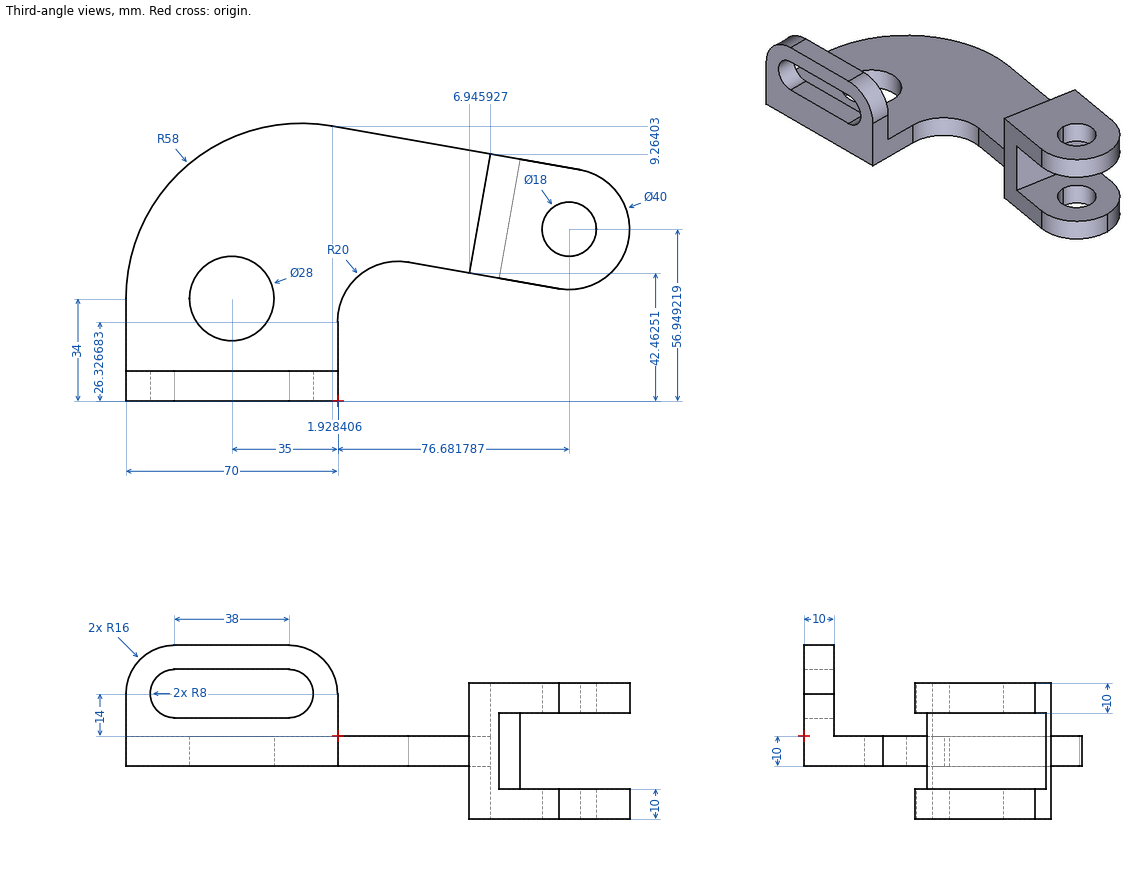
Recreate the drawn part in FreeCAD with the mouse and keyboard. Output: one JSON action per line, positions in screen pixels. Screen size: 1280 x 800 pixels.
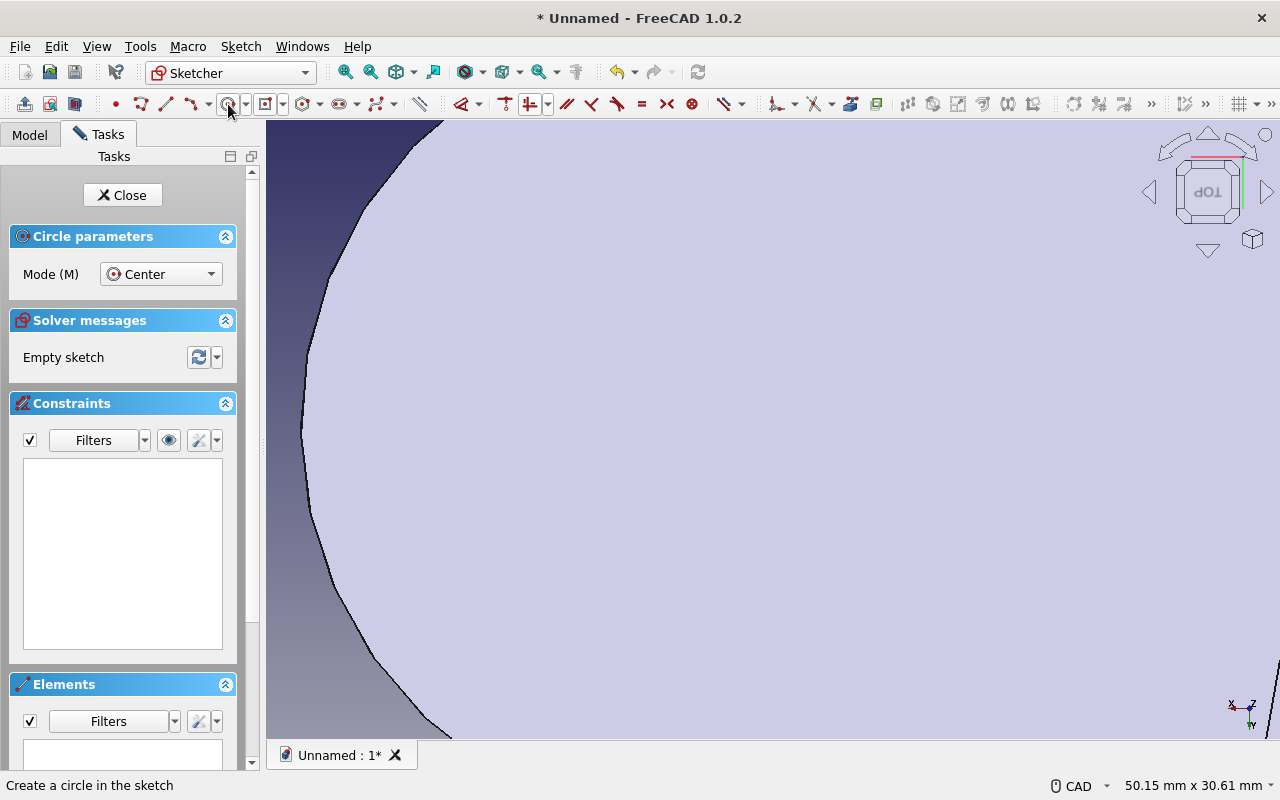
{"action": "left_click", "coordinate": [705, 426]}
{"action": "left_click", "coordinate": [834, 297]}
{"action": "key", "text": "Escape"}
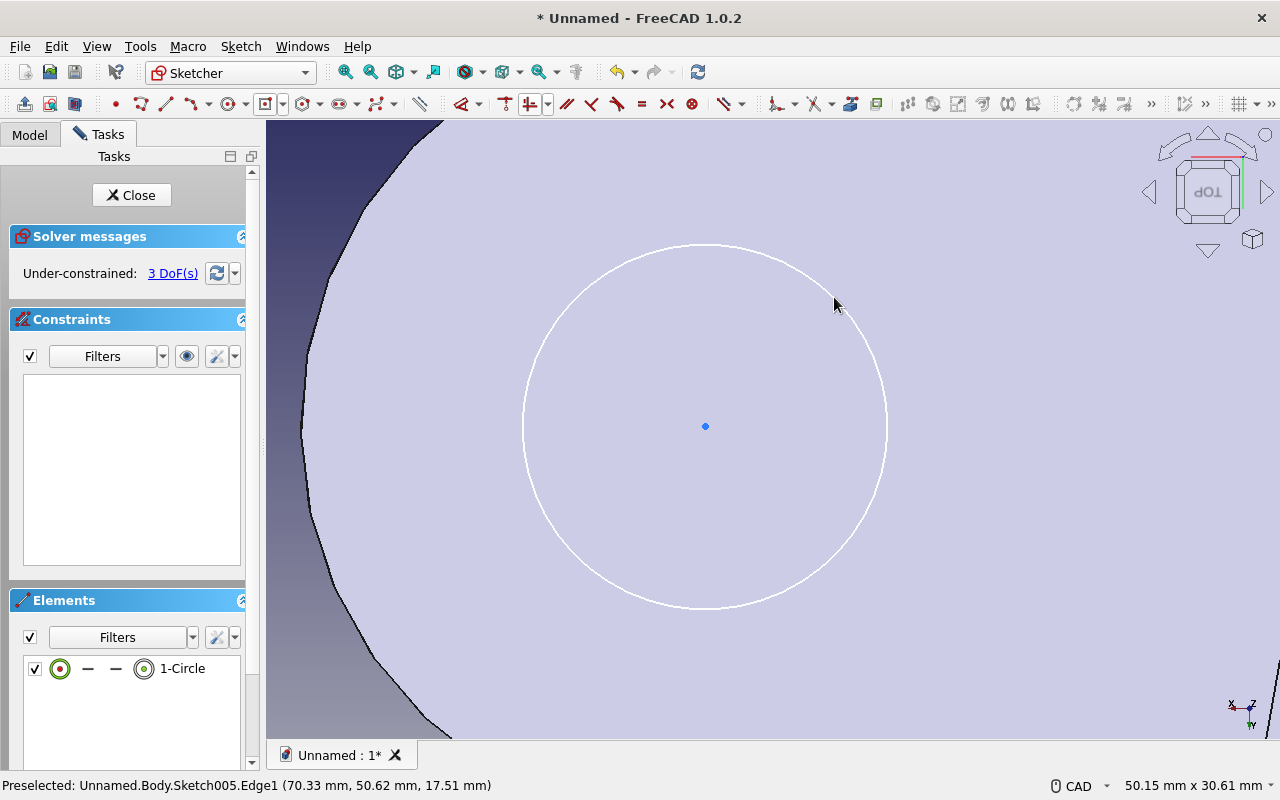
{"action": "left_click", "coordinate": [460, 104]}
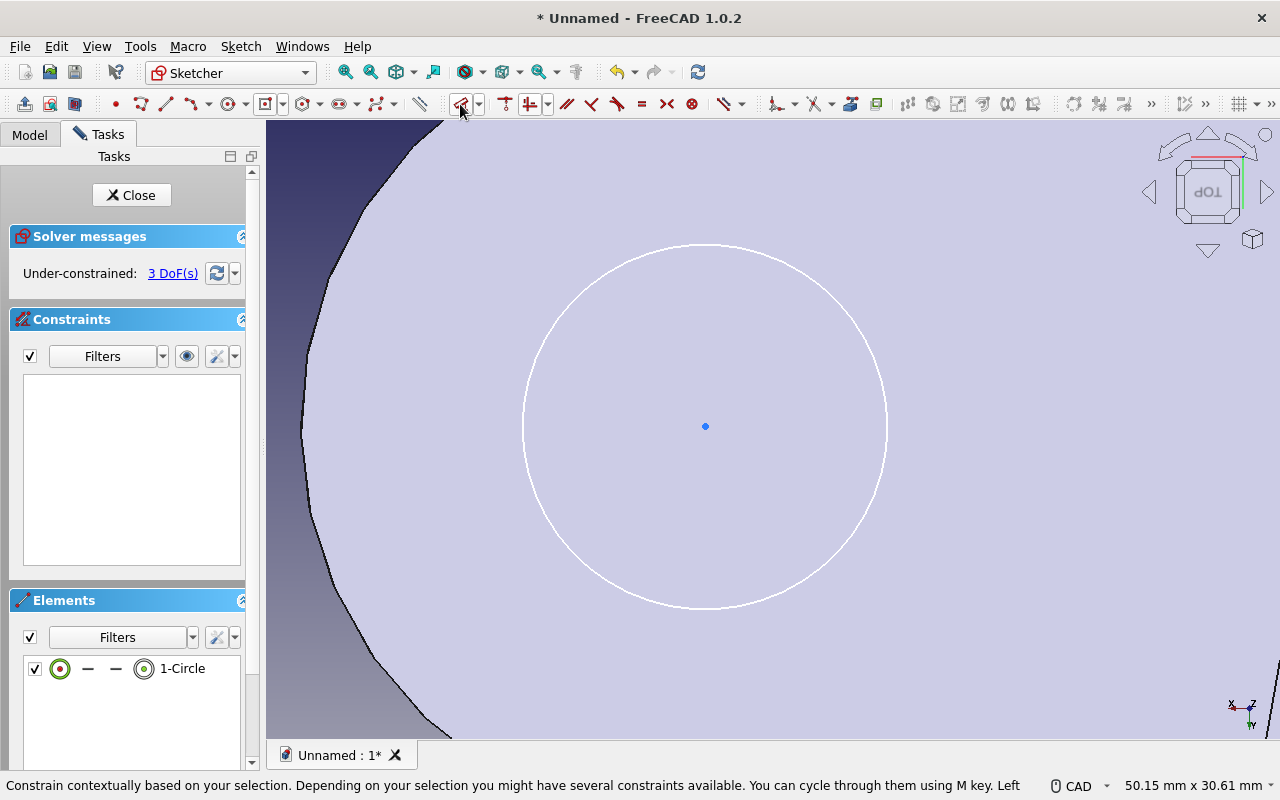
{"action": "left_click", "coordinate": [834, 298]}
{"action": "left_click", "coordinate": [857, 275]}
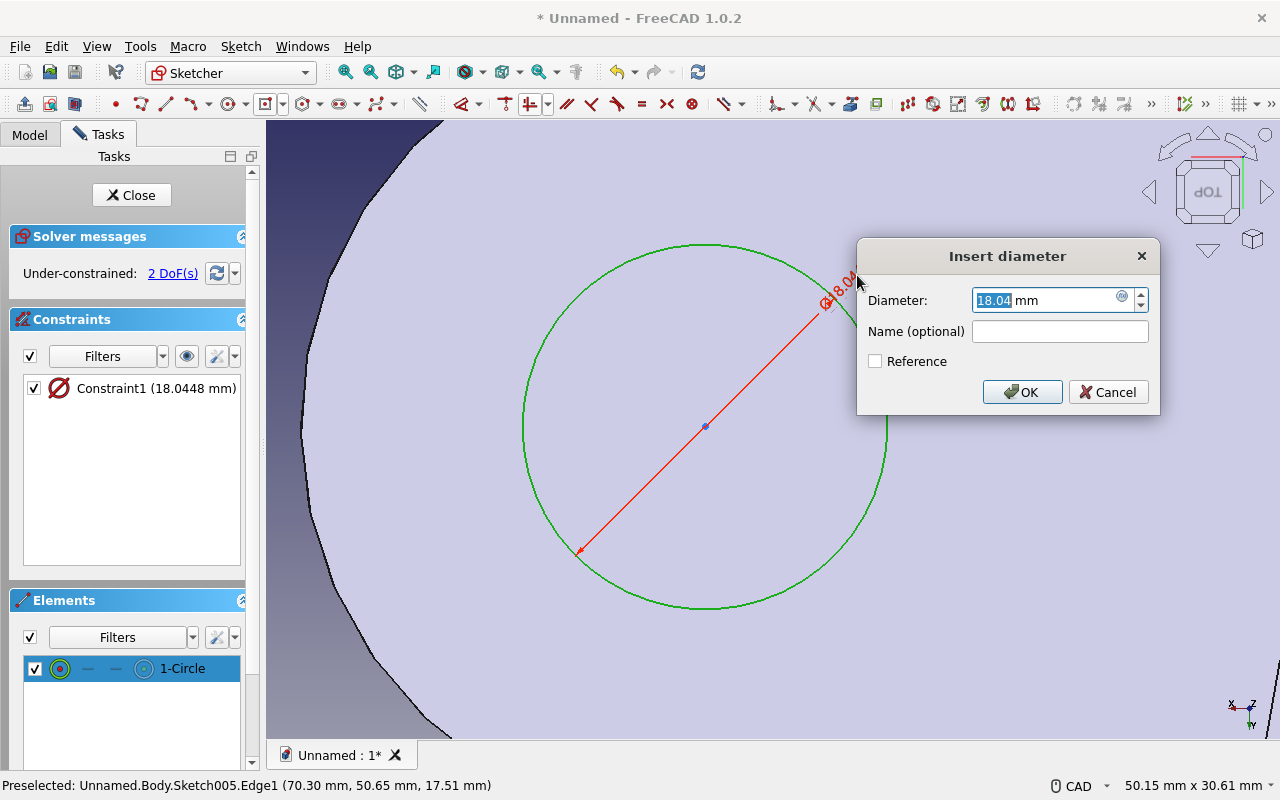
{"action": "type", "text": "18"}
{"action": "key", "text": "Return"}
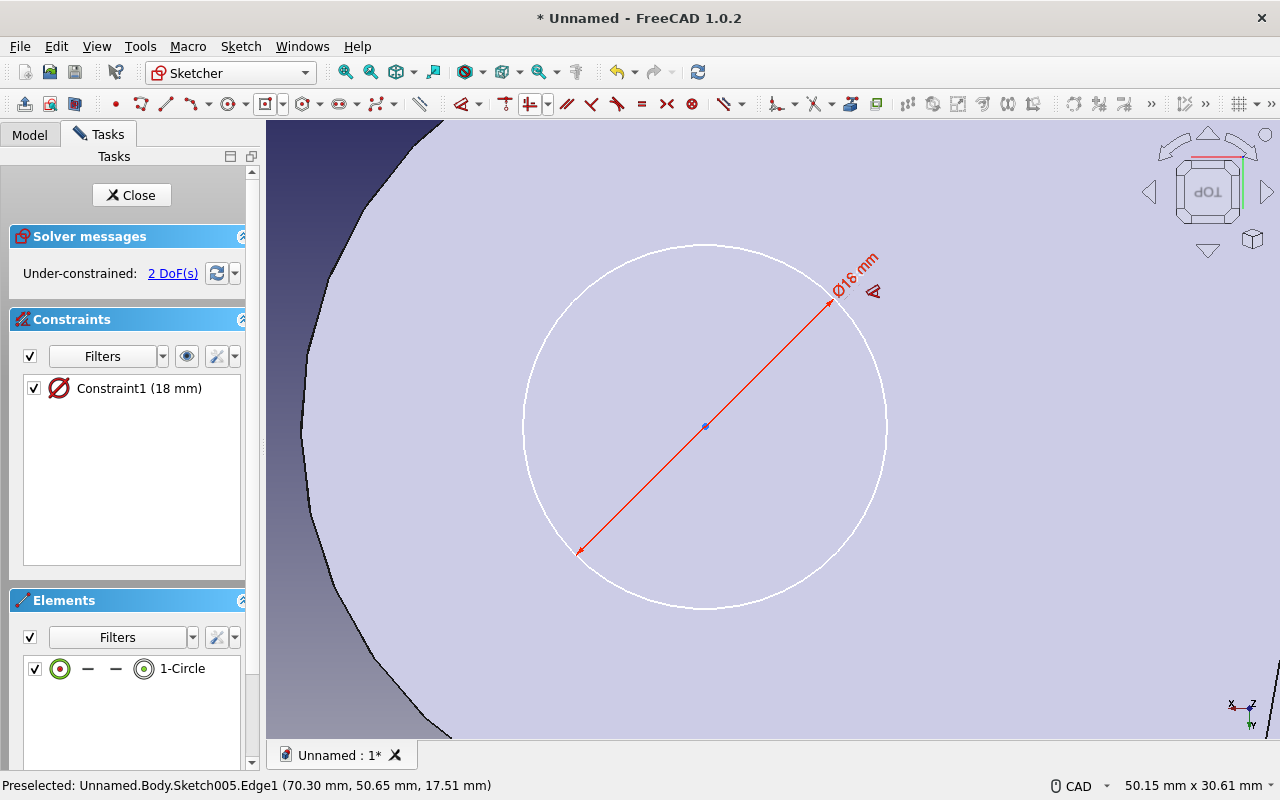
{"action": "left_click", "coordinate": [705, 427]}
{"action": "left_click", "coordinate": [910, 461]}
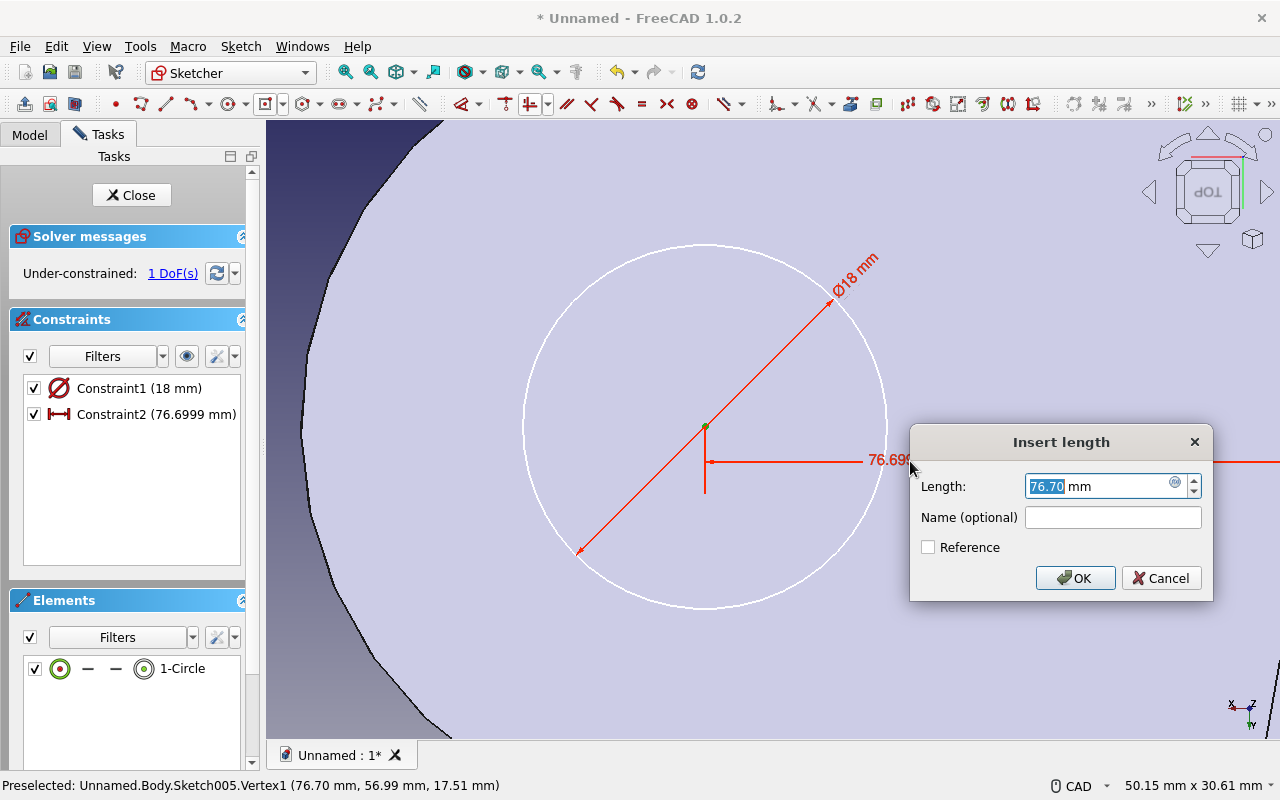
{"action": "type", "text": "76.681787"}
{"action": "key", "text": "Return"}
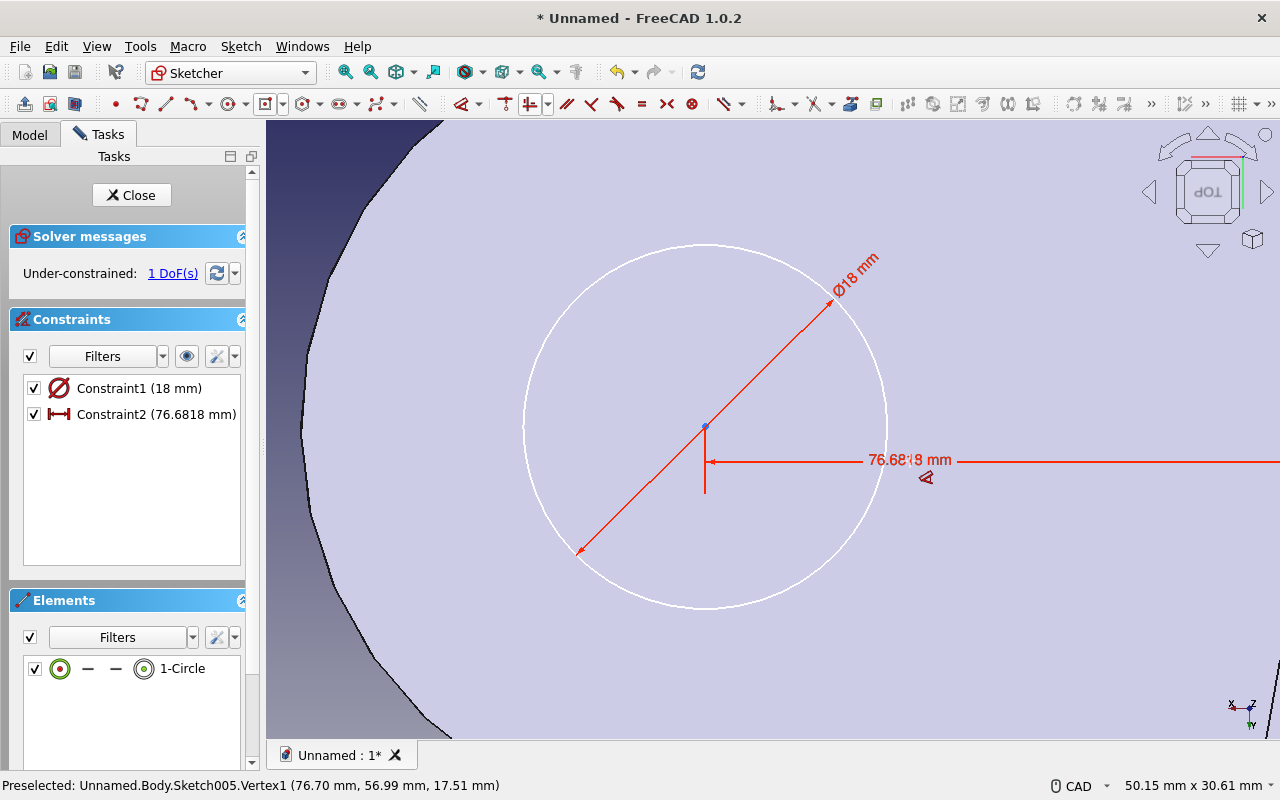
{"action": "left_click", "coordinate": [705, 427]}
{"action": "left_click", "coordinate": [671, 288]}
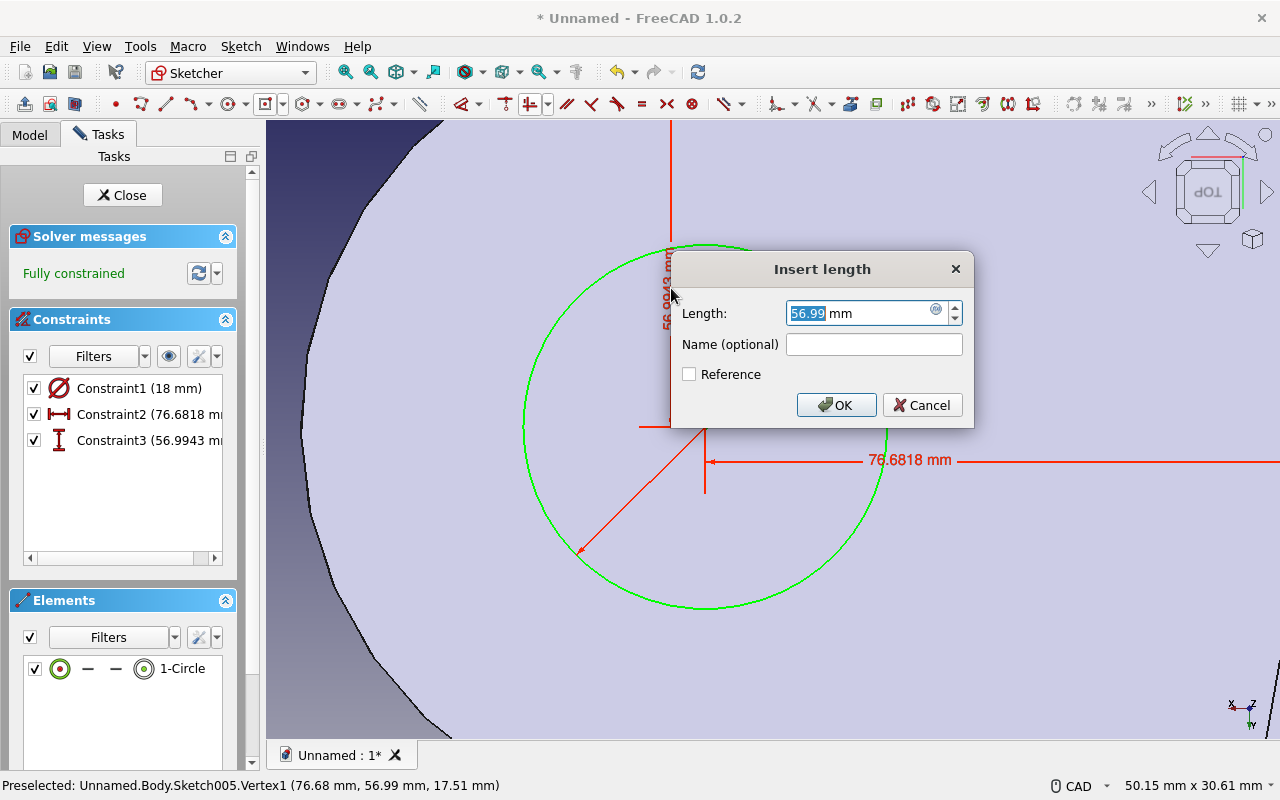
{"action": "type", "text": "56.949219"}
{"action": "key", "text": "Return"}
{"action": "key", "text": "Escape"}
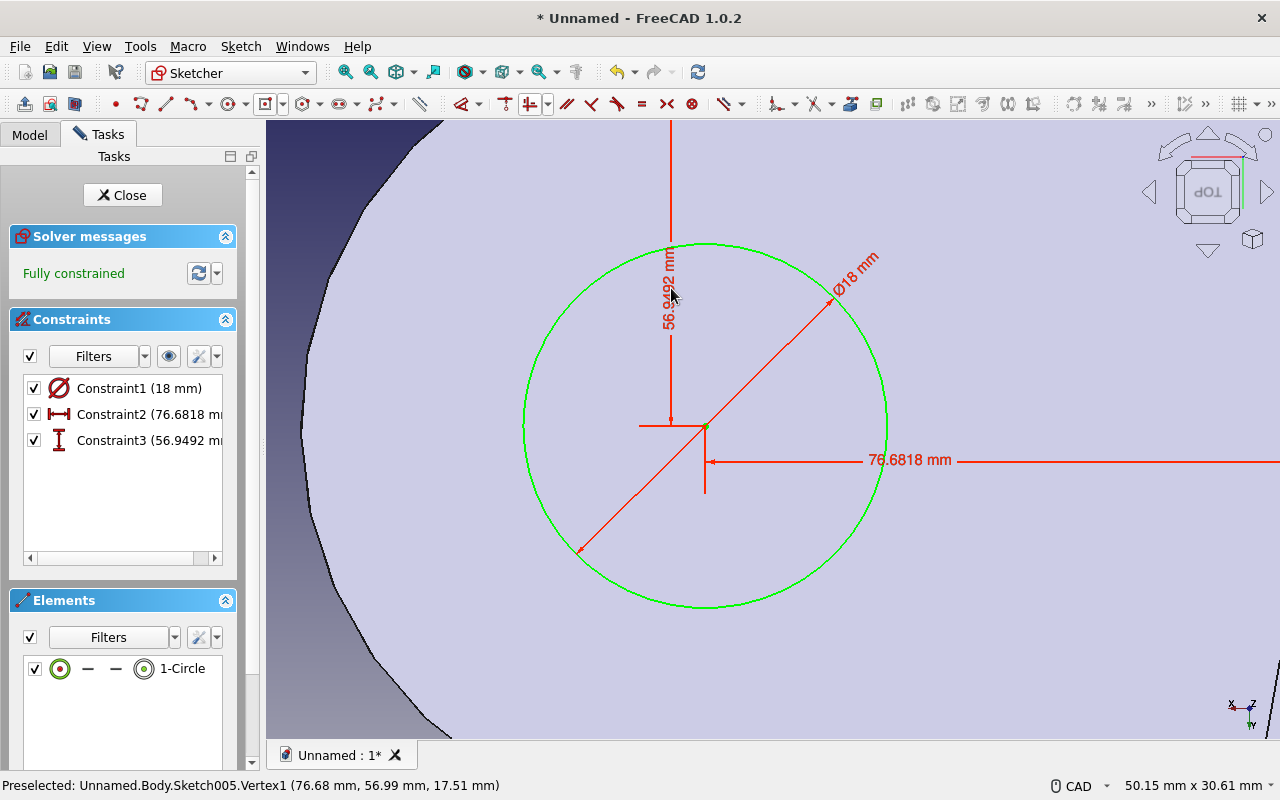
{"action": "left_click", "coordinate": [123, 195]}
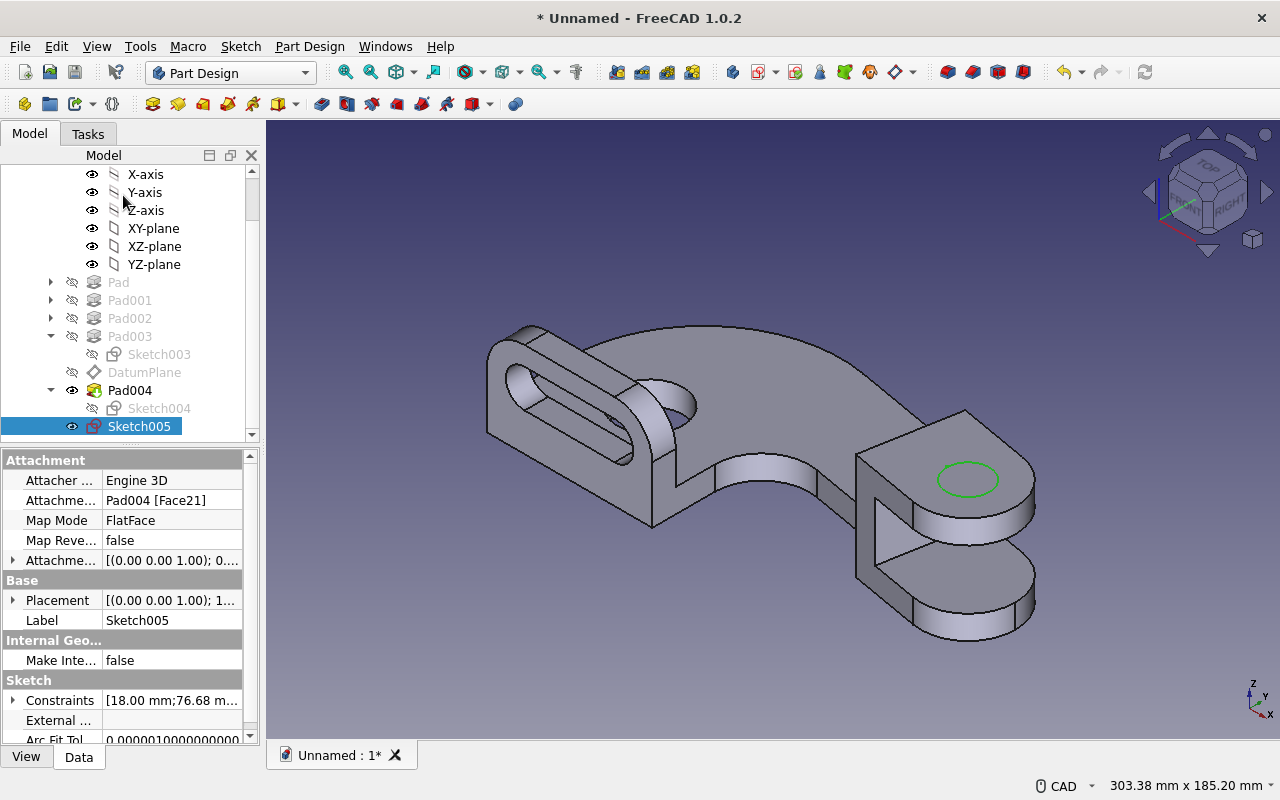
{"action": "left_click", "coordinate": [322, 104]}